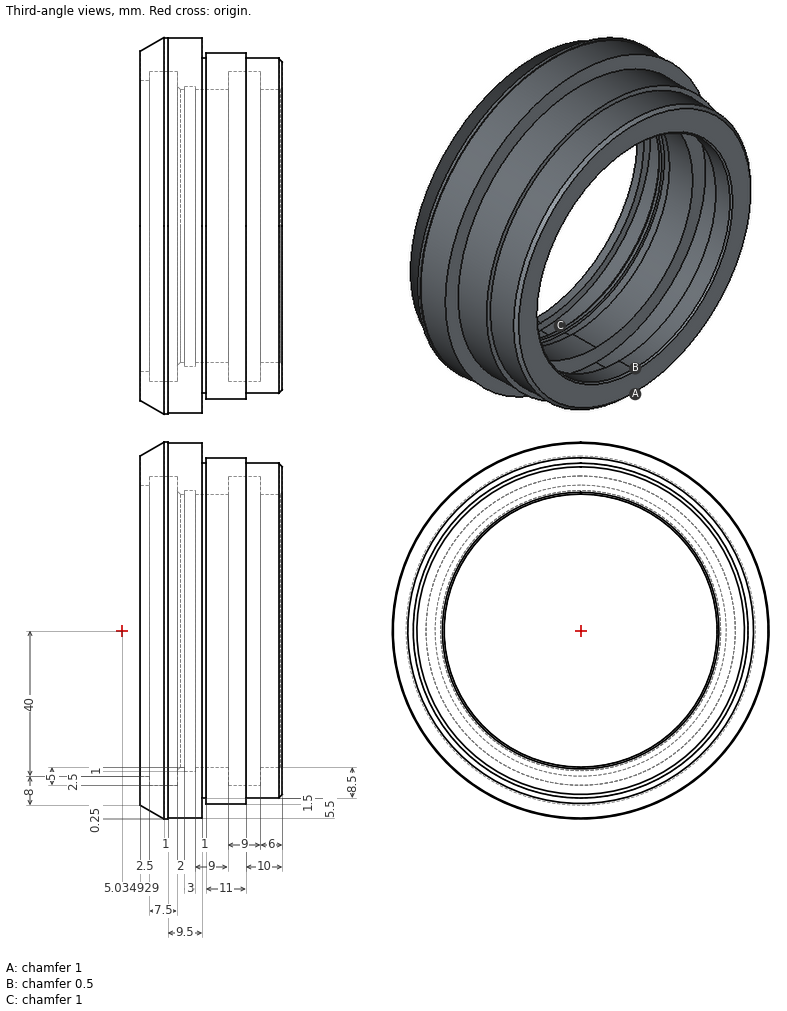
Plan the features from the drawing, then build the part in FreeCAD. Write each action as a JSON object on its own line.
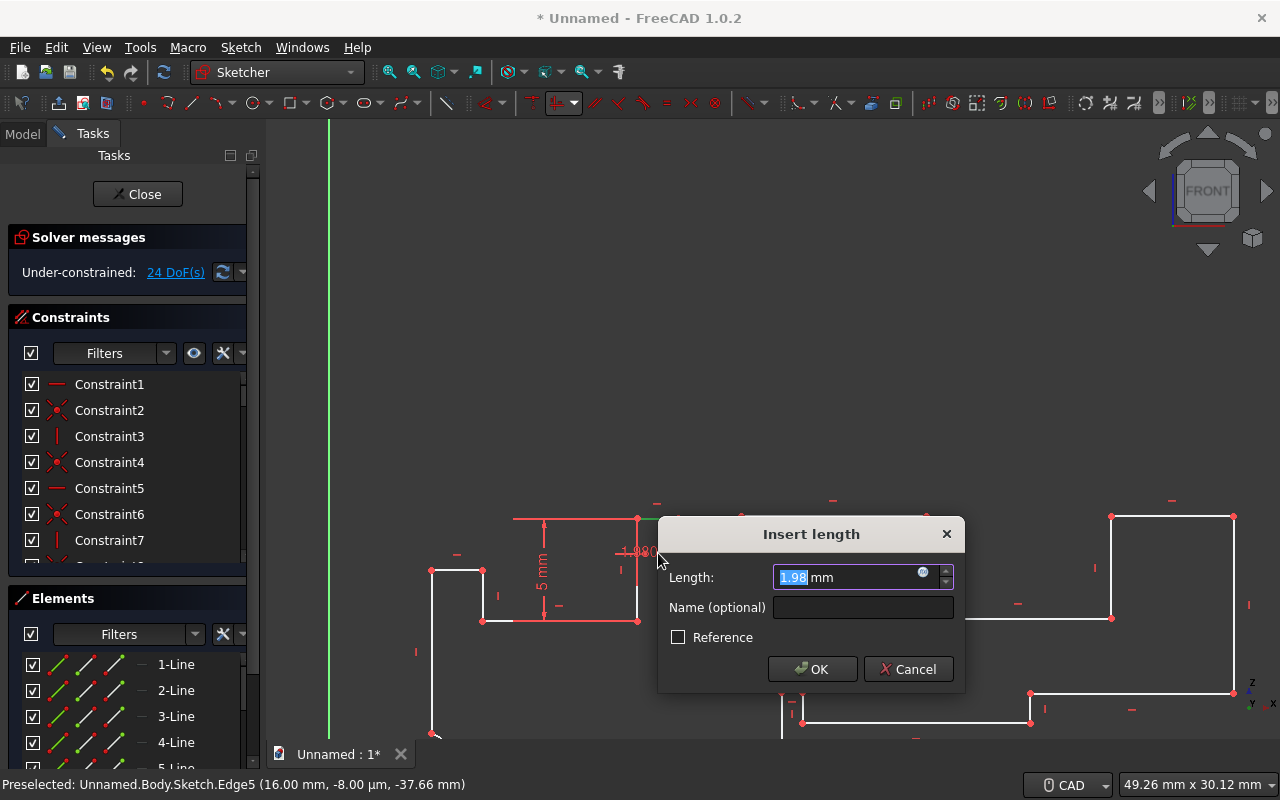
{"action": "type", "text": "2"}
{"action": "key", "text": "Return"}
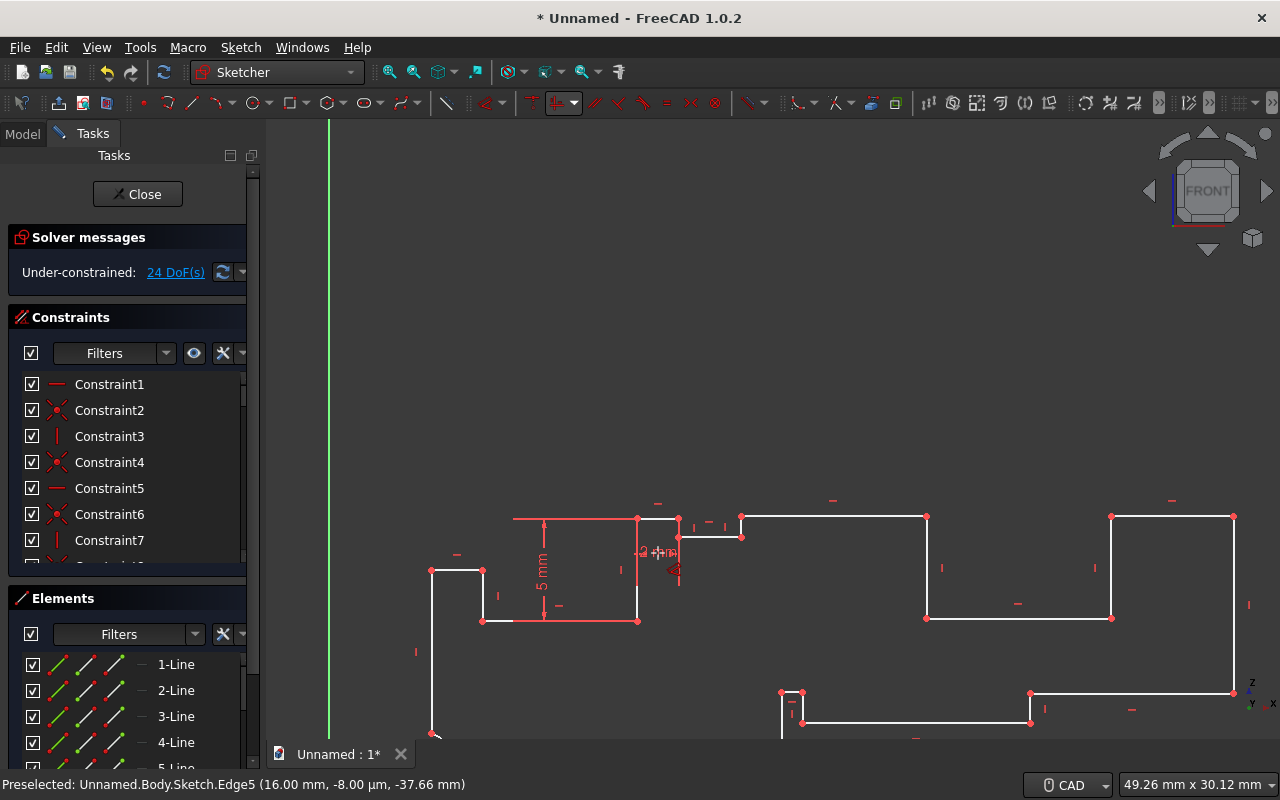
{"action": "scroll", "coordinate": [679, 528], "scroll_direction": "up", "scroll_amount": 4}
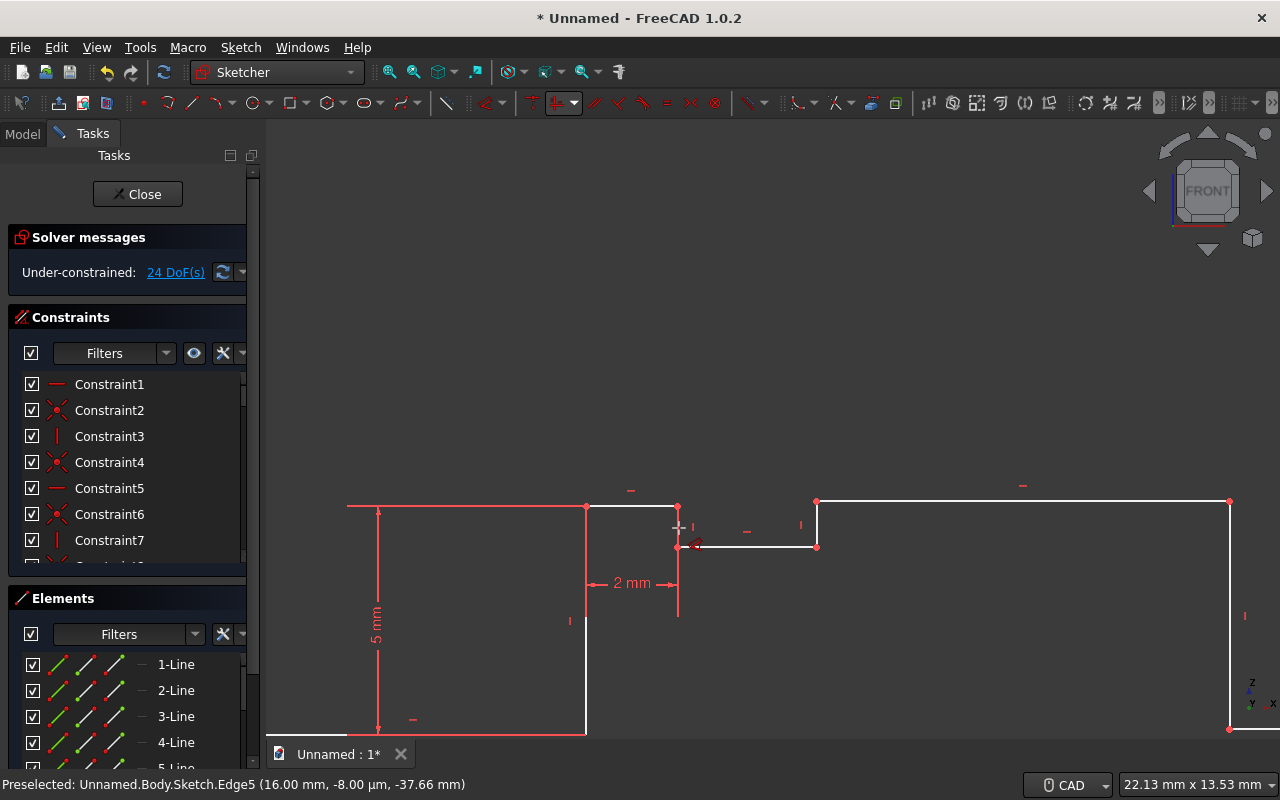
{"action": "left_click", "coordinate": [678, 527]}
{"action": "left_click", "coordinate": [644, 527]}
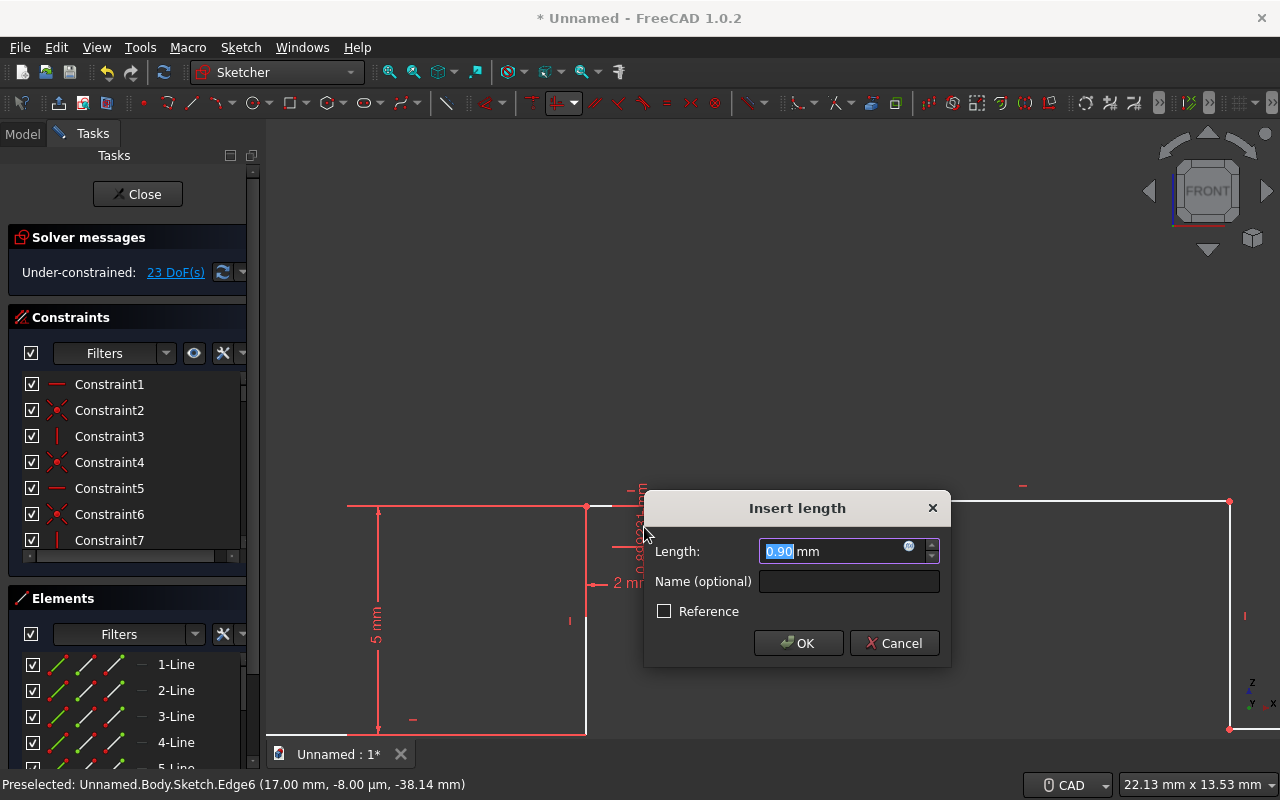
{"action": "type", "text": "1"}
{"action": "key", "text": "Return"}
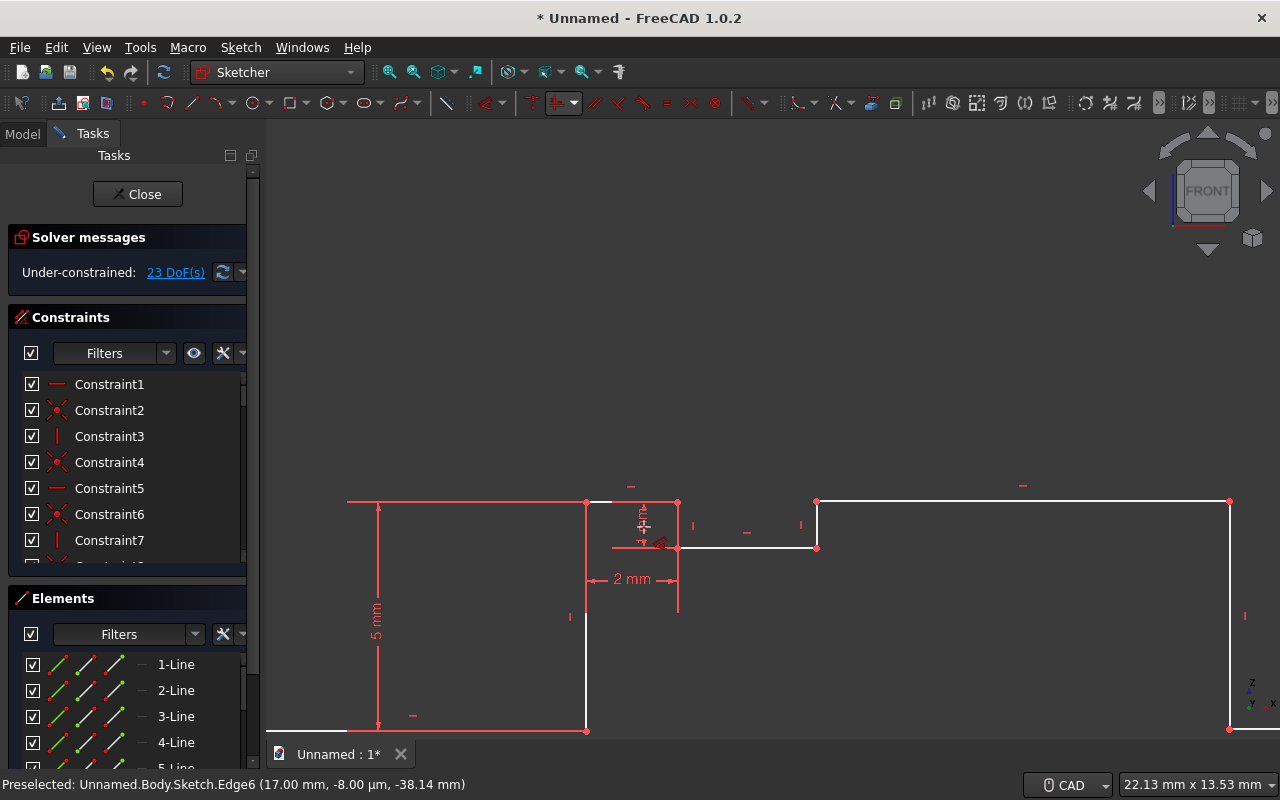
{"action": "scroll", "coordinate": [664, 521], "scroll_direction": "down", "scroll_amount": 9}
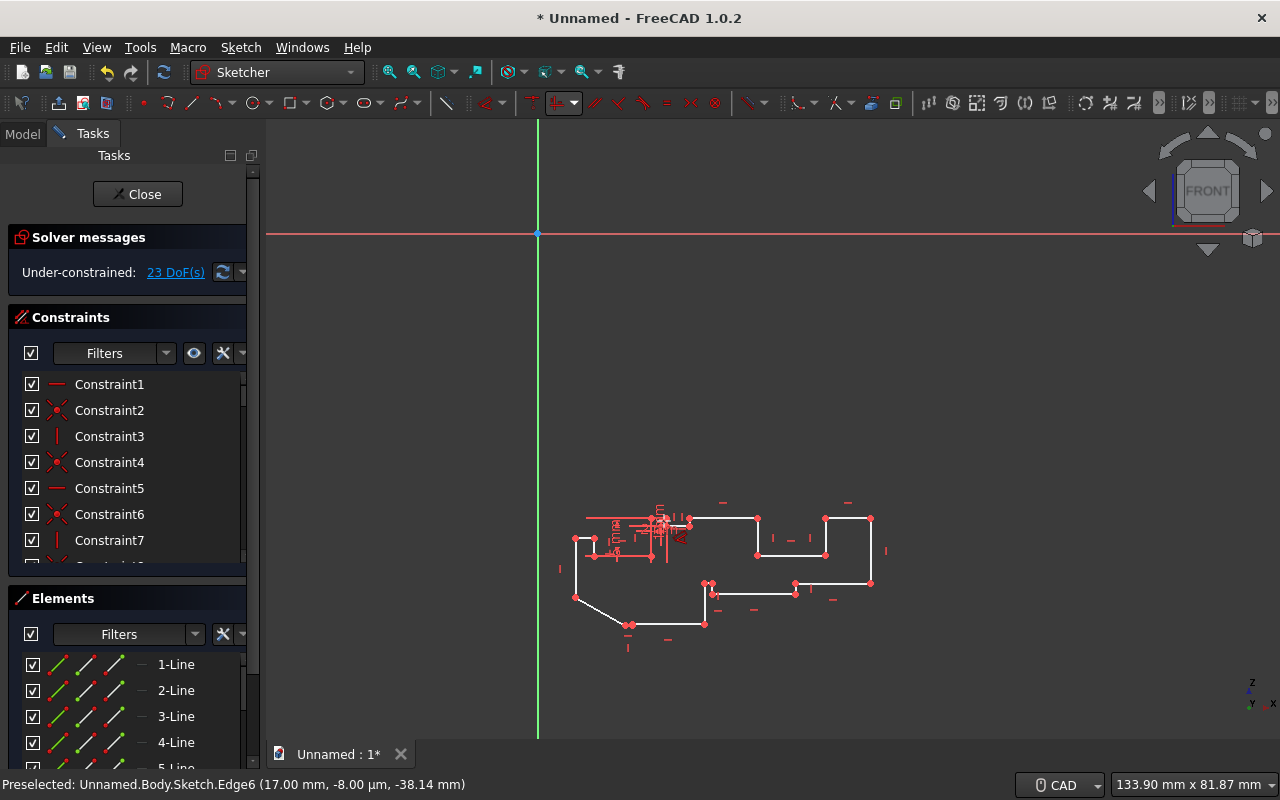
{"action": "scroll", "coordinate": [673, 526], "scroll_direction": "up", "scroll_amount": 4}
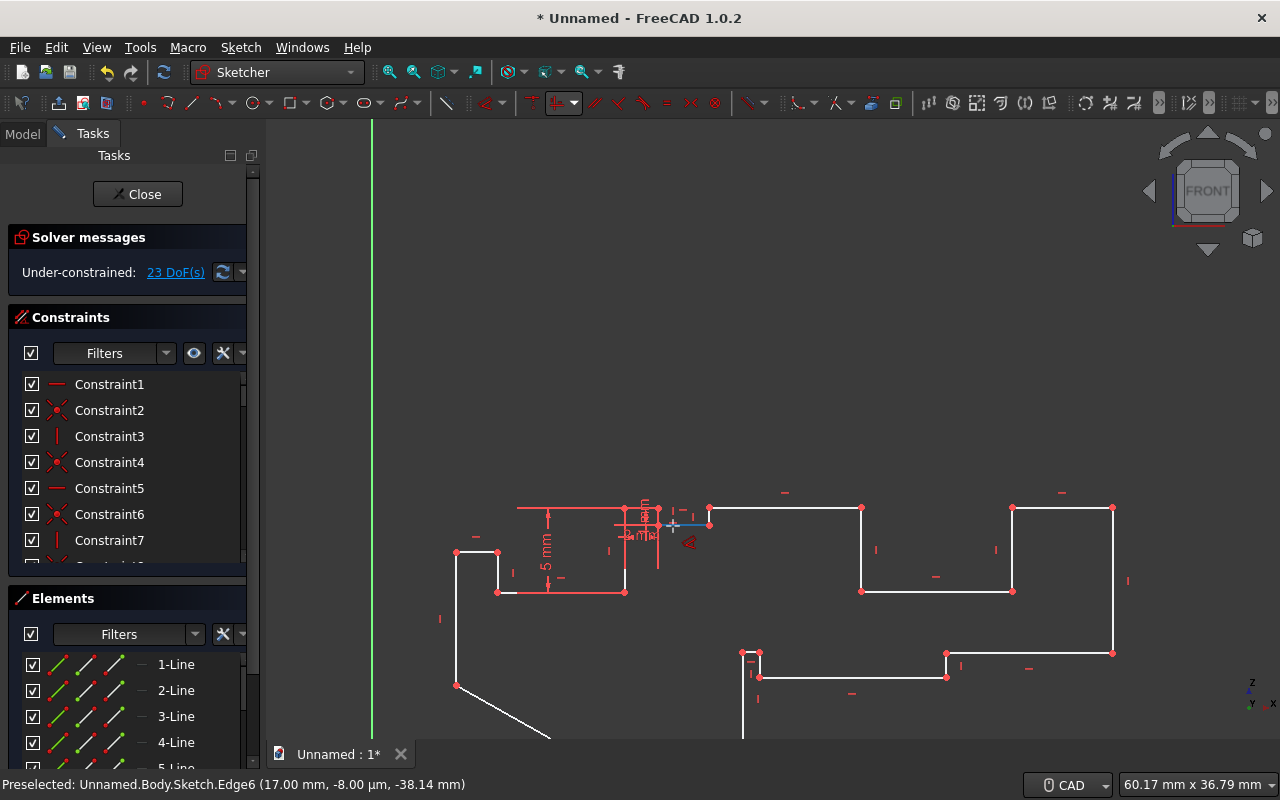
{"action": "left_click", "coordinate": [674, 525]}
{"action": "left_click", "coordinate": [684, 559]}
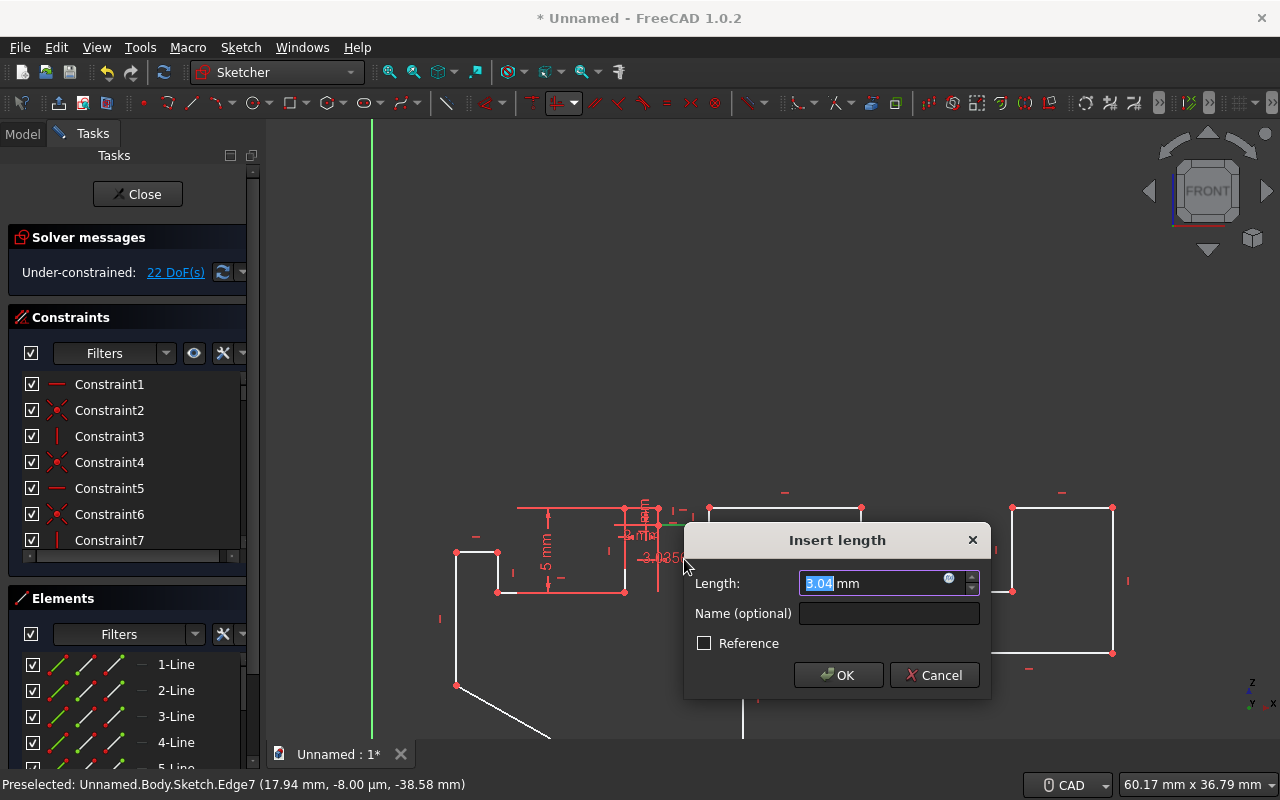
{"action": "type", "text": "3"}
{"action": "key", "text": "Return"}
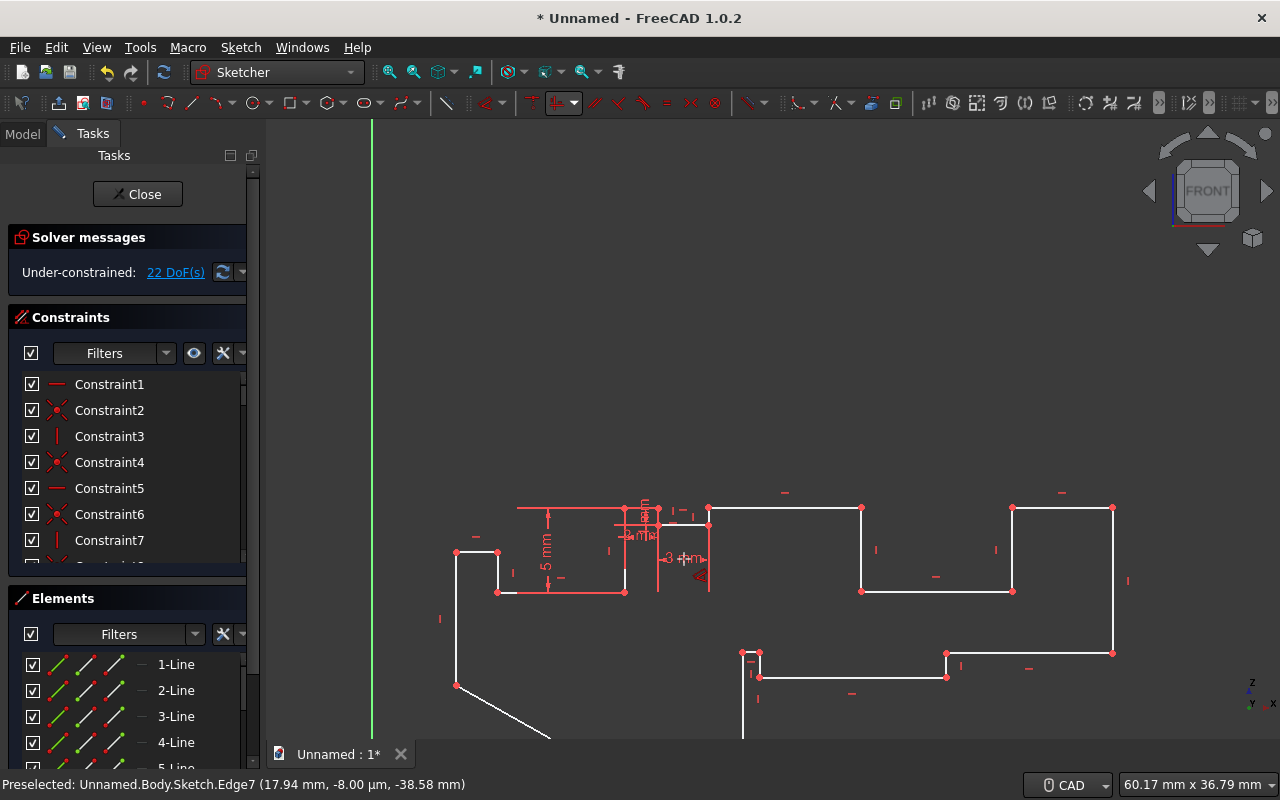
{"action": "scroll", "coordinate": [709, 517], "scroll_direction": "up", "scroll_amount": 5}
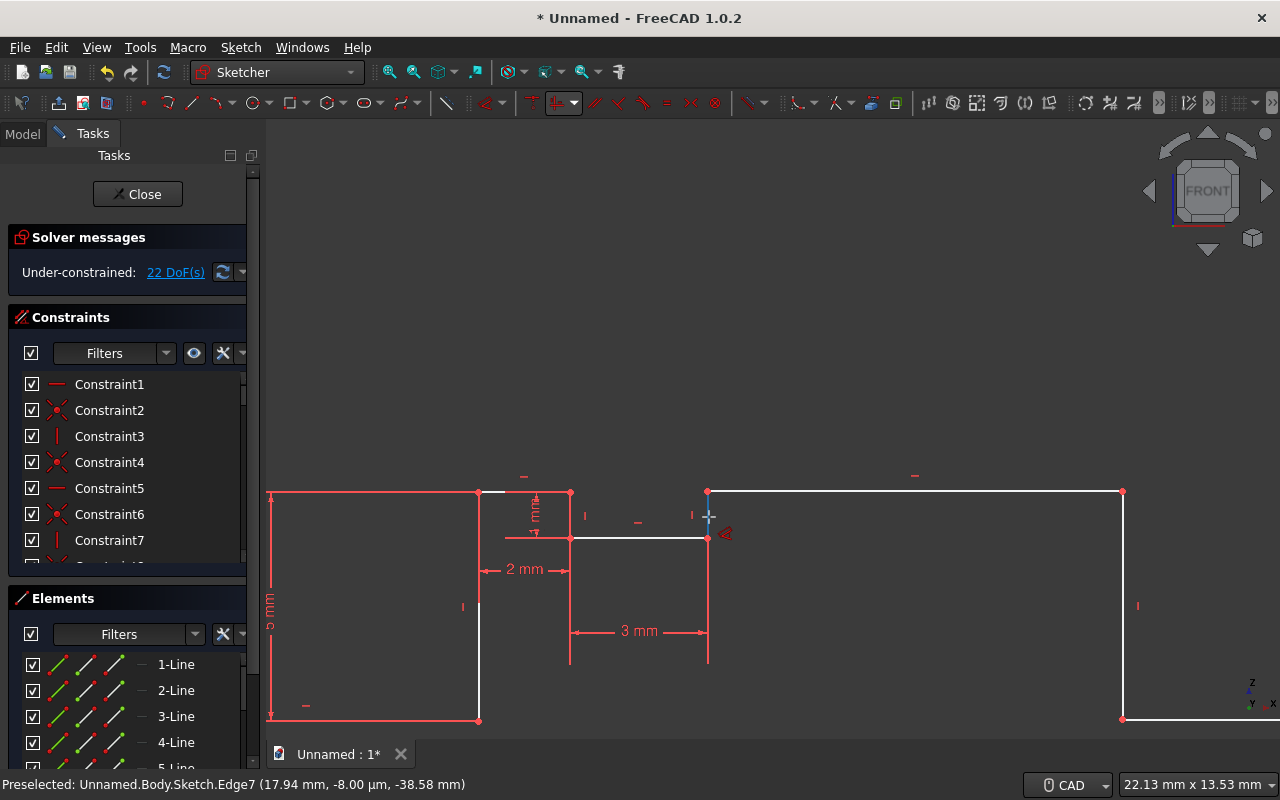
{"action": "left_click", "coordinate": [708, 515]}
{"action": "left_click", "coordinate": [674, 515]}